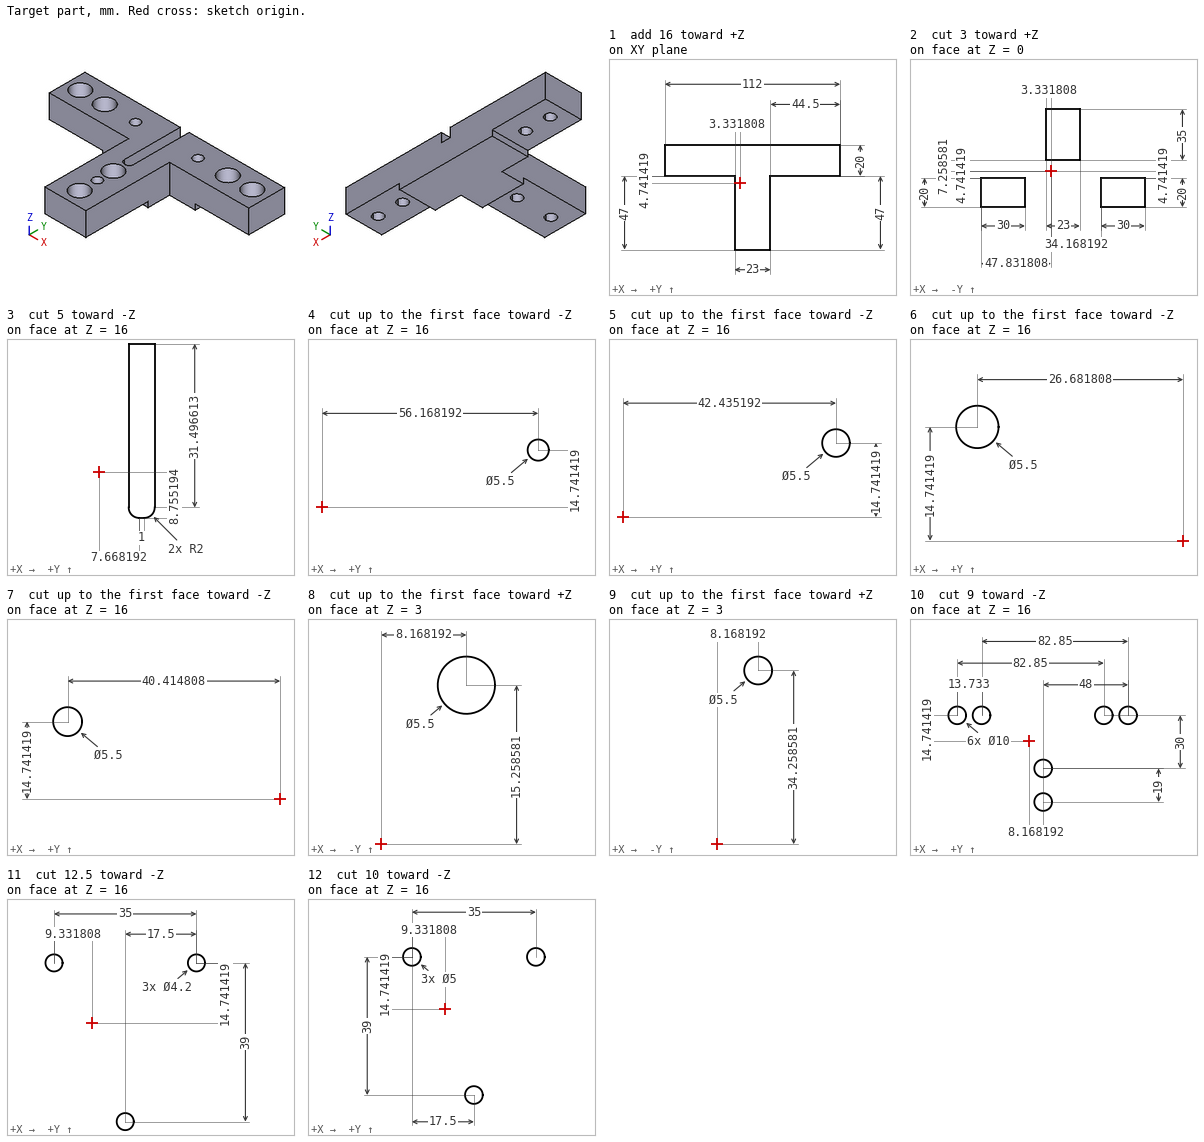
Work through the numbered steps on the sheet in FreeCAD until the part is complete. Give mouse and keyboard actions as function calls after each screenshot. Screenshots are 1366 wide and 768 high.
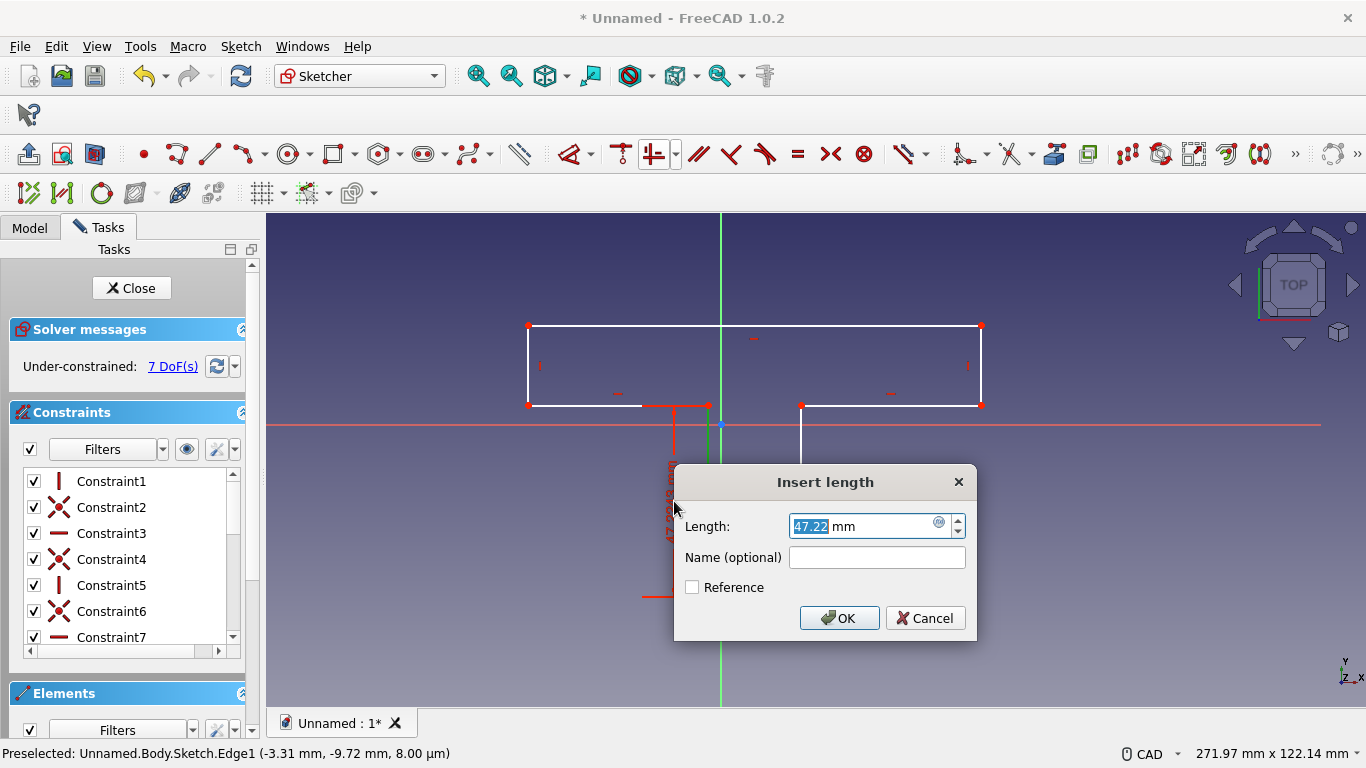
text(47)
key(Return)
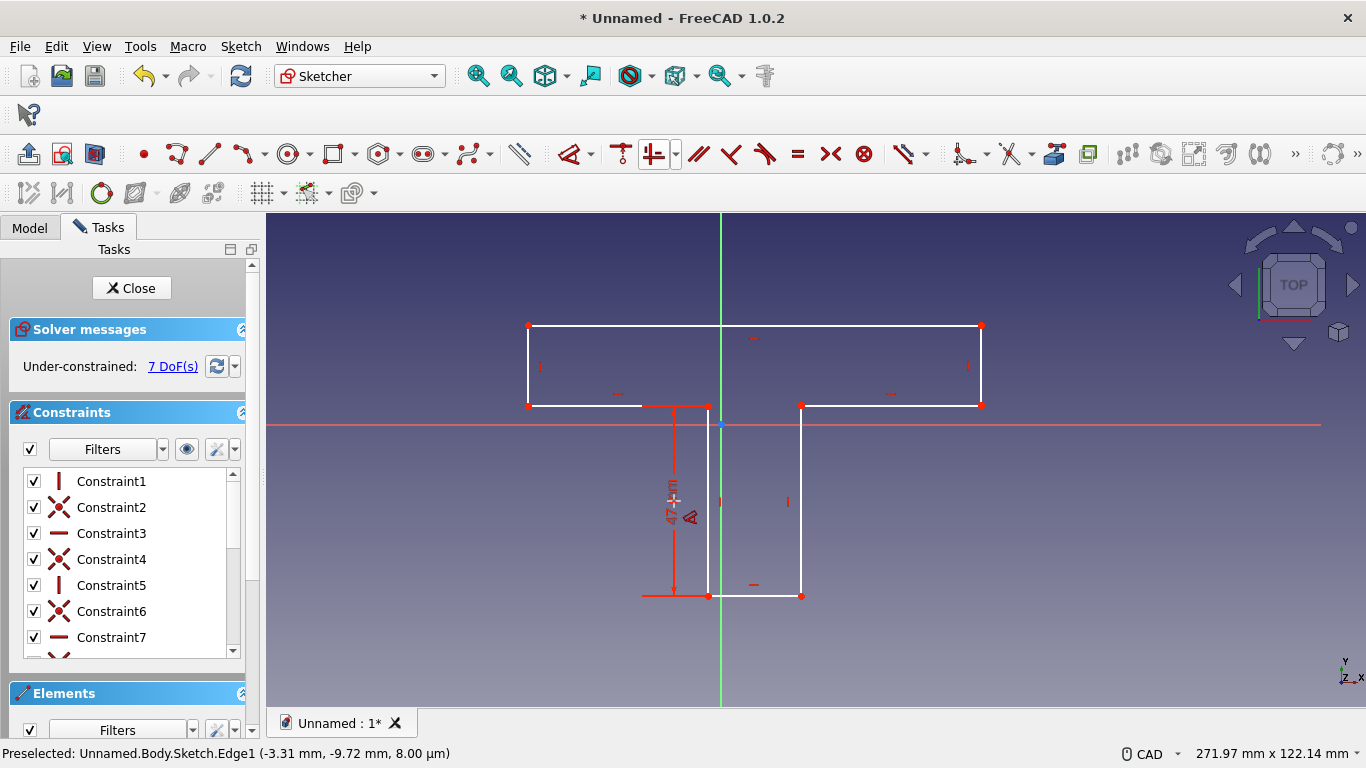
click(736, 596)
click(755, 630)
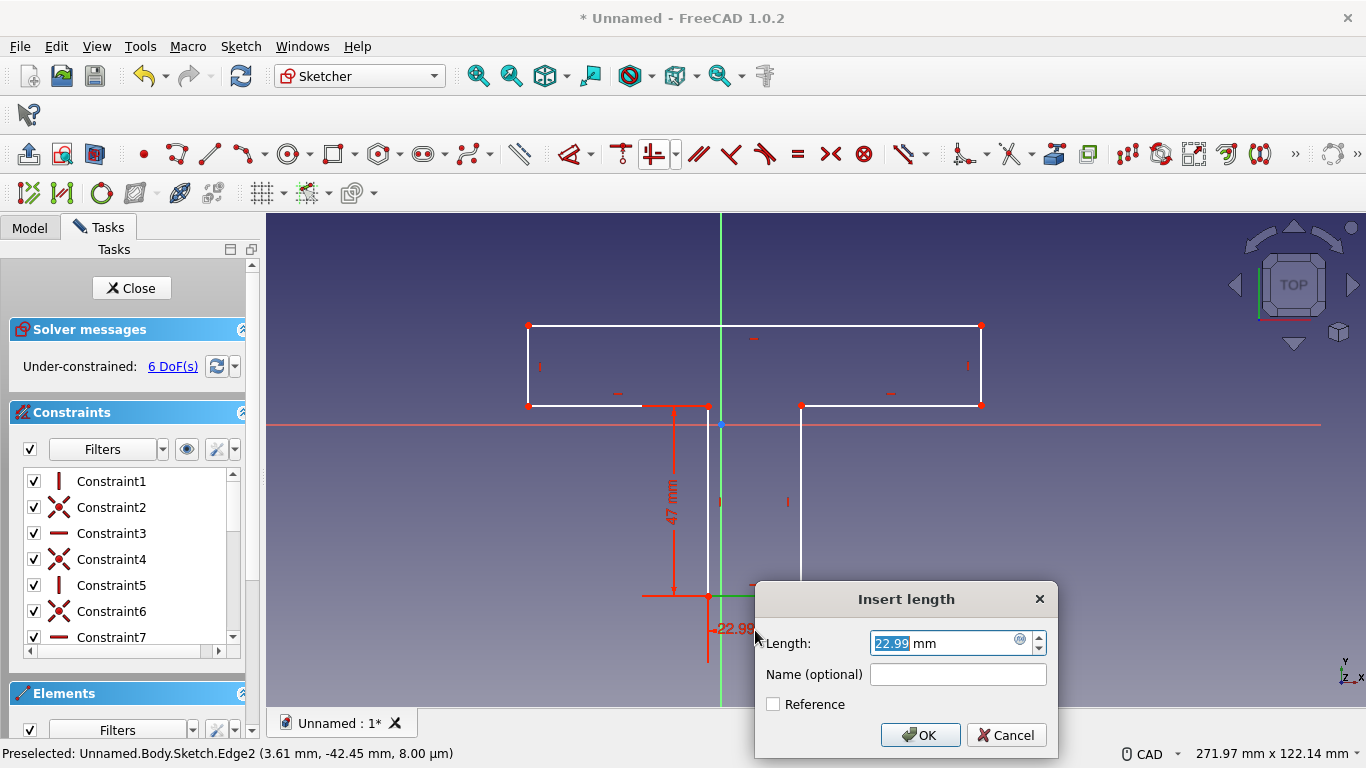
text(23)
key(Return)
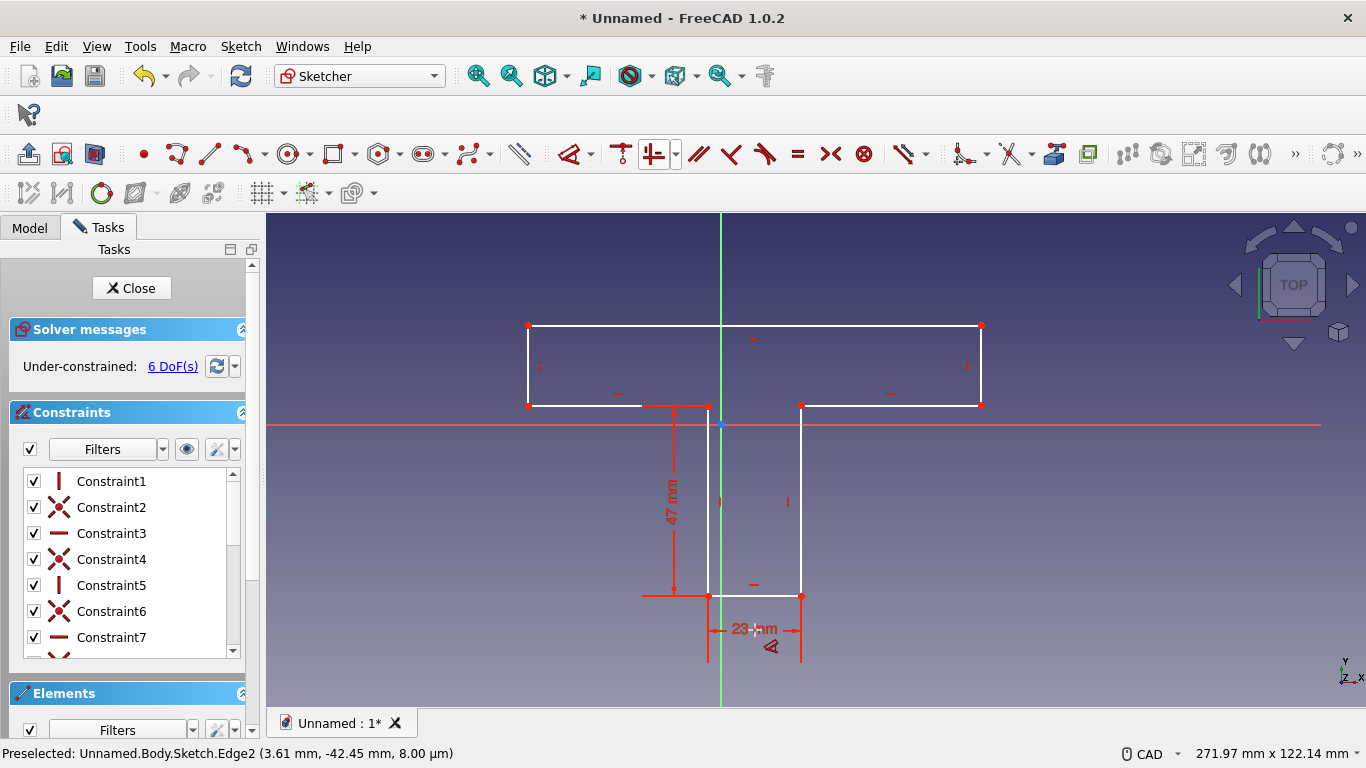
click(801, 539)
click(835, 501)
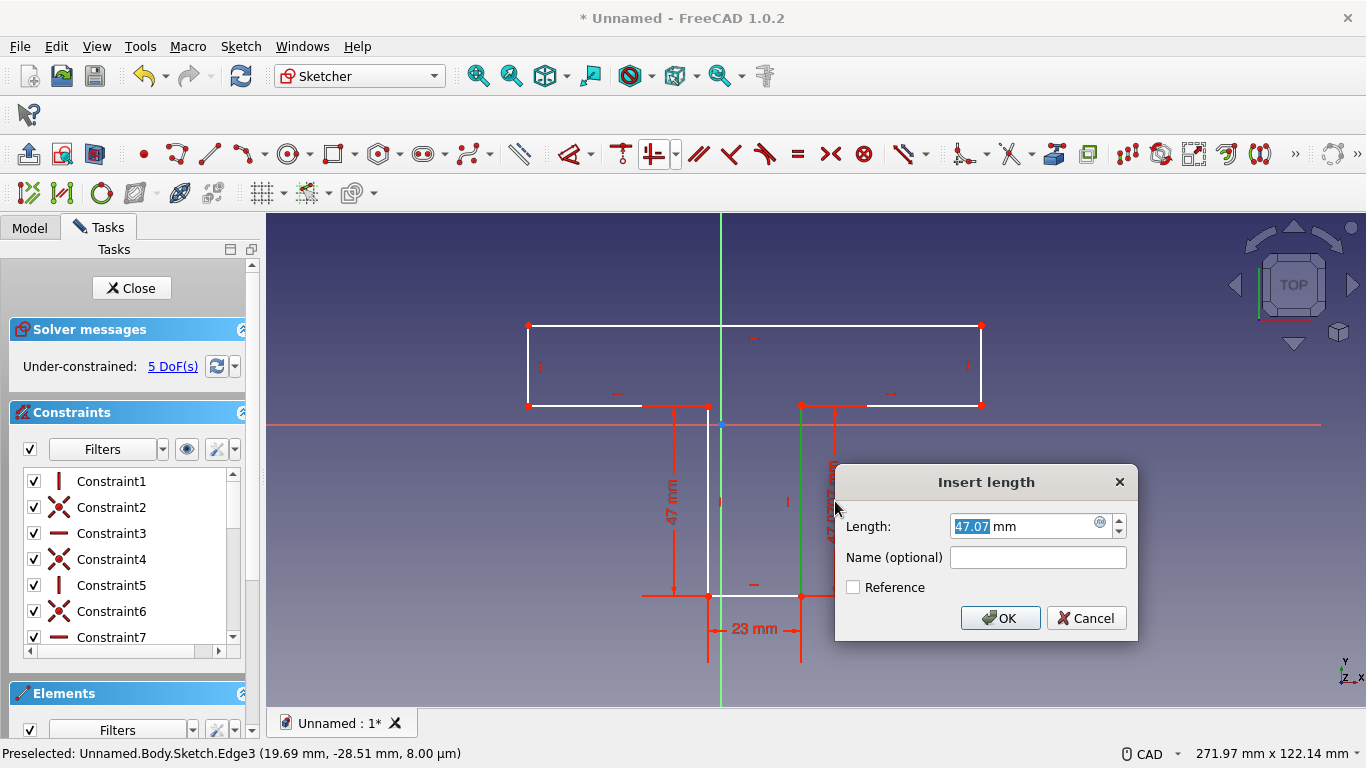
text(47)
key(Return)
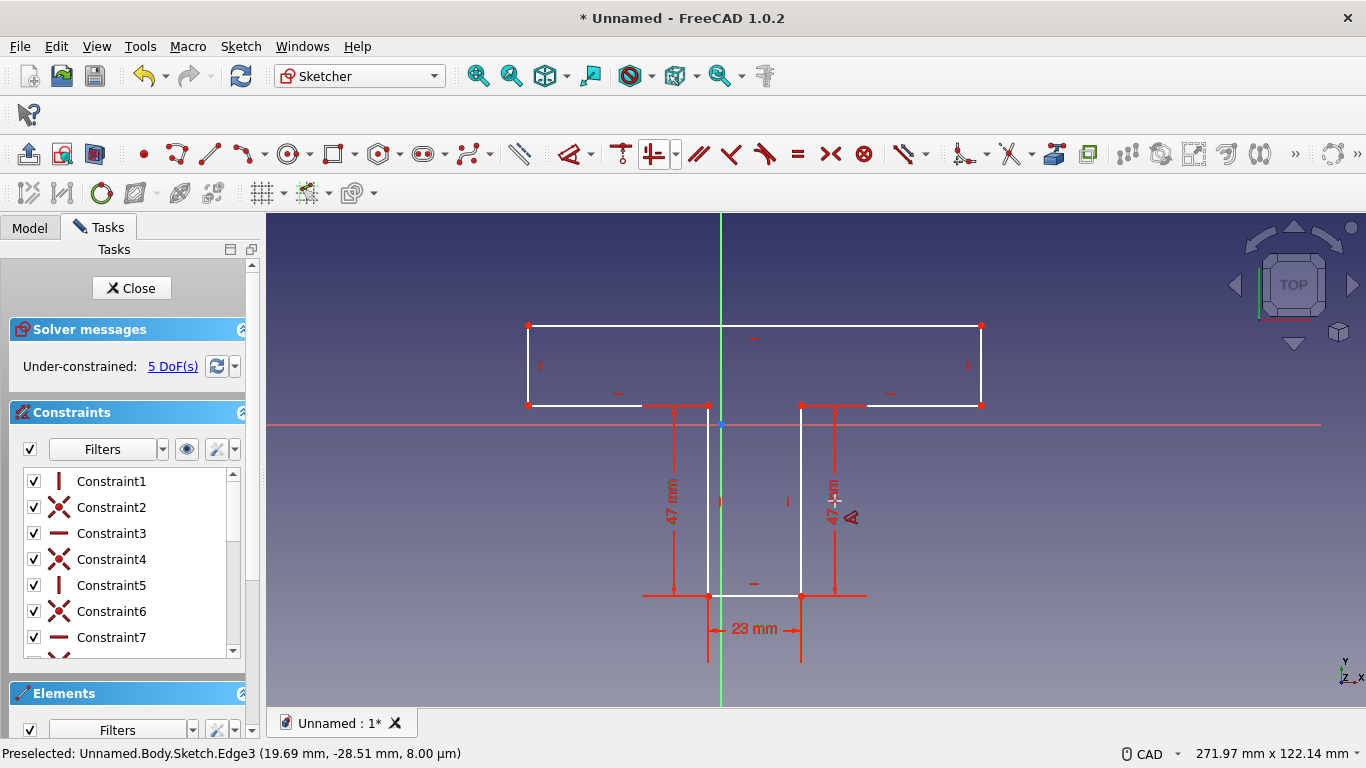
click(981, 382)
click(1015, 366)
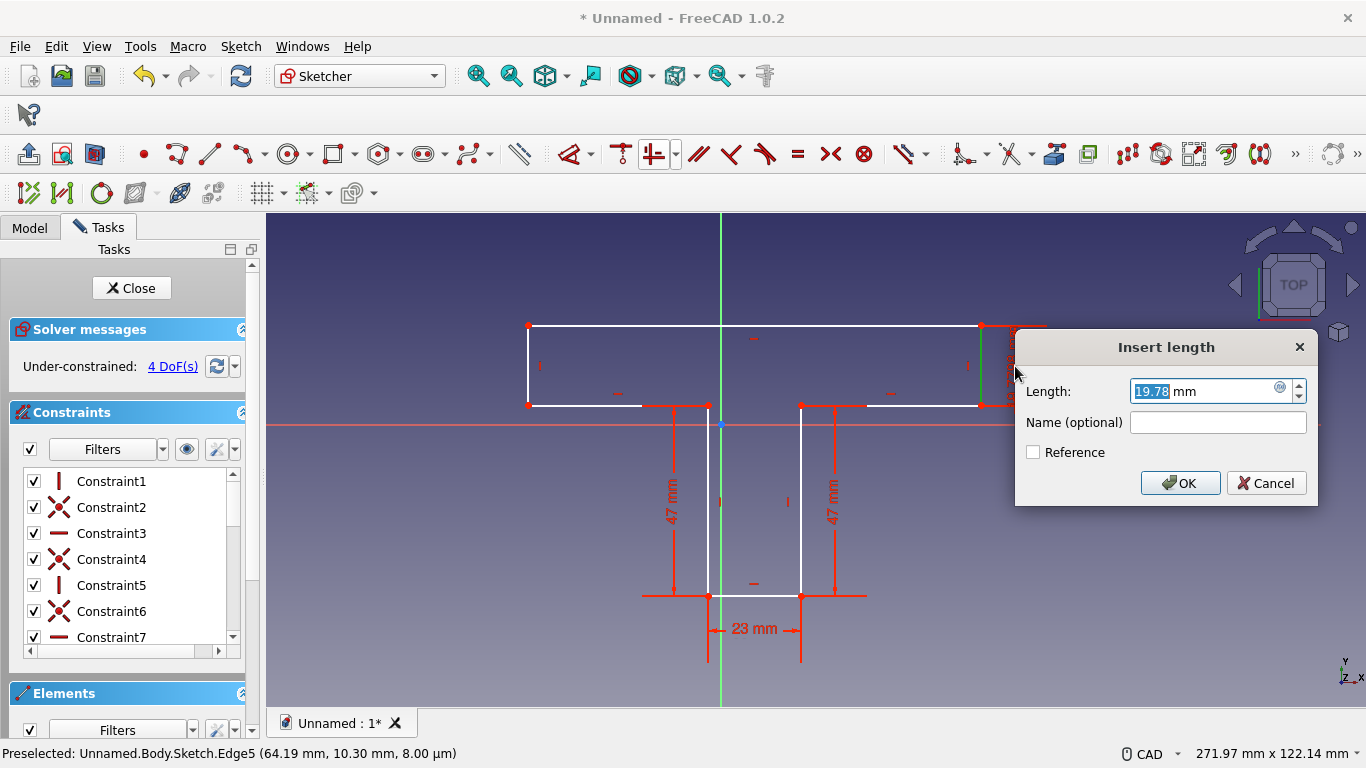
text(20)
key(Return)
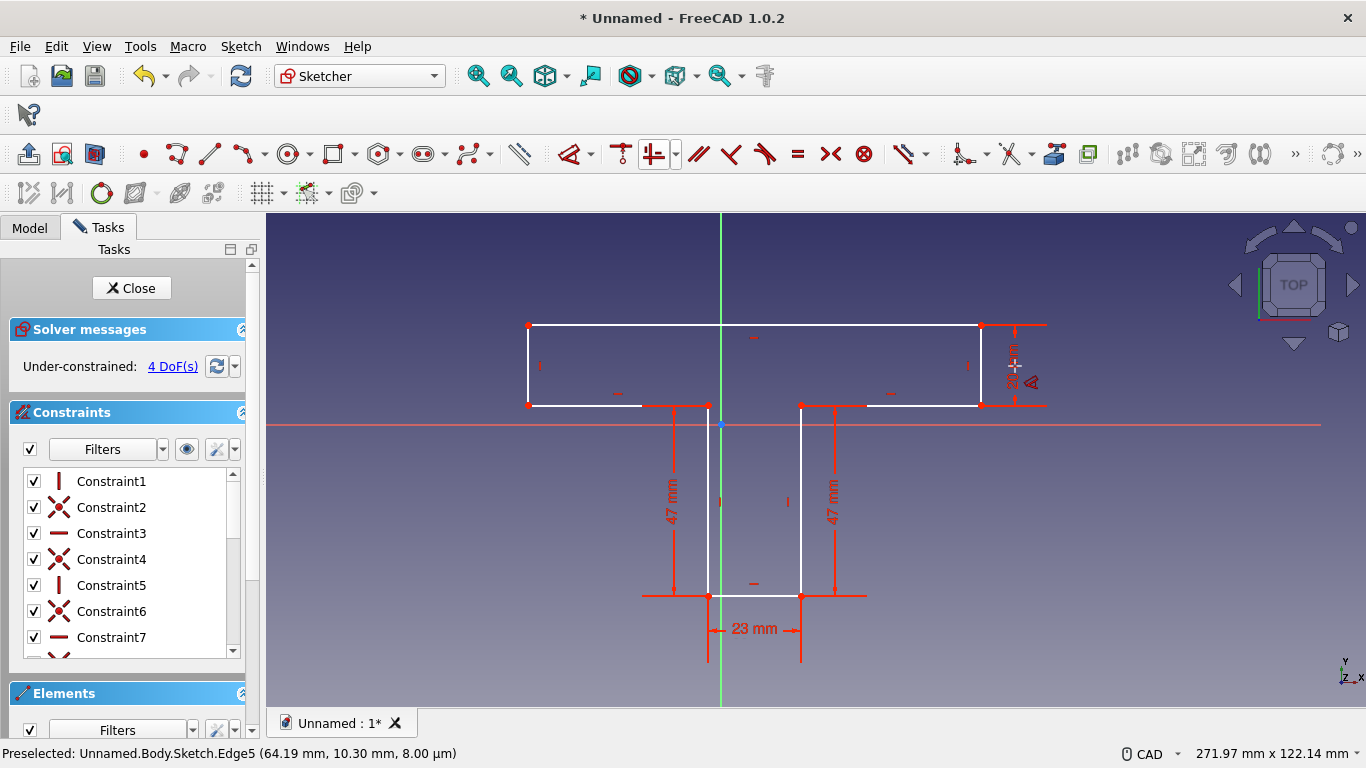
click(845, 325)
click(754, 291)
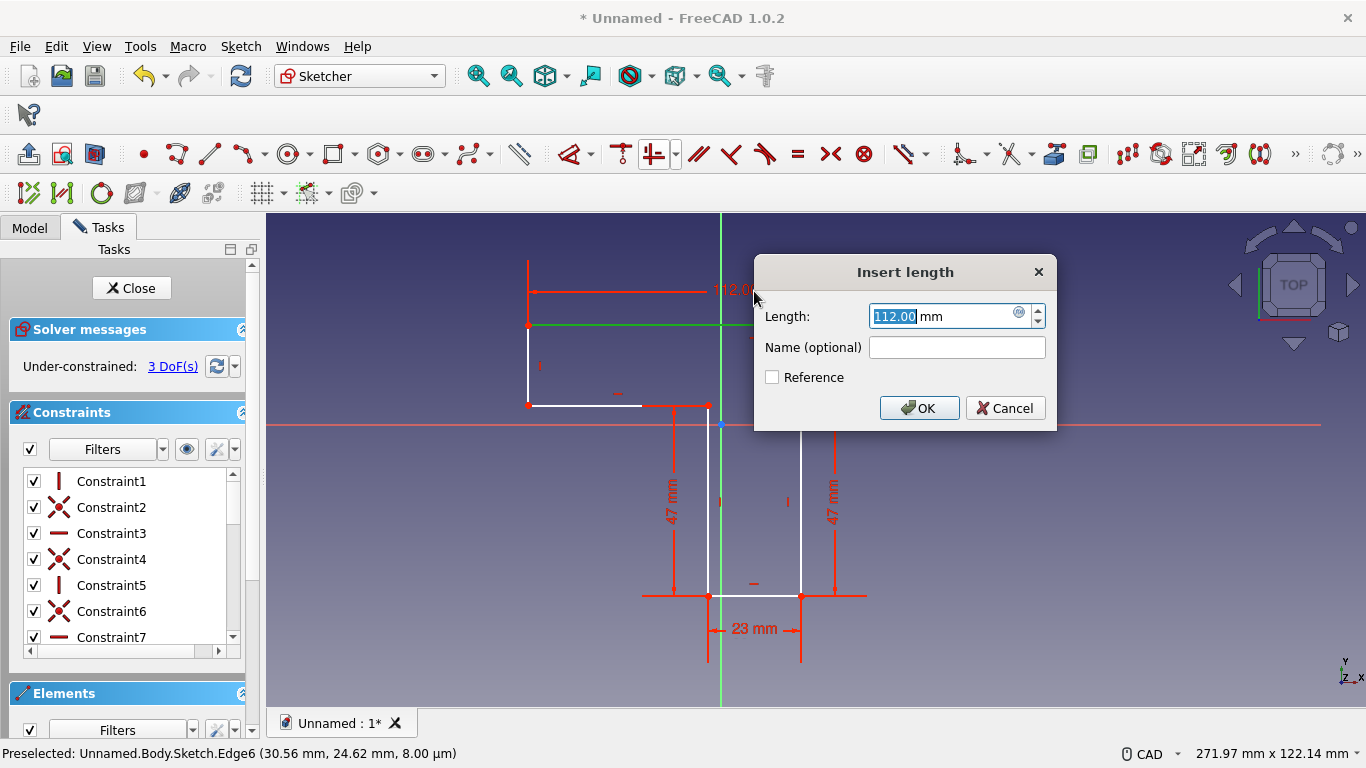
text(112)
key(Return)